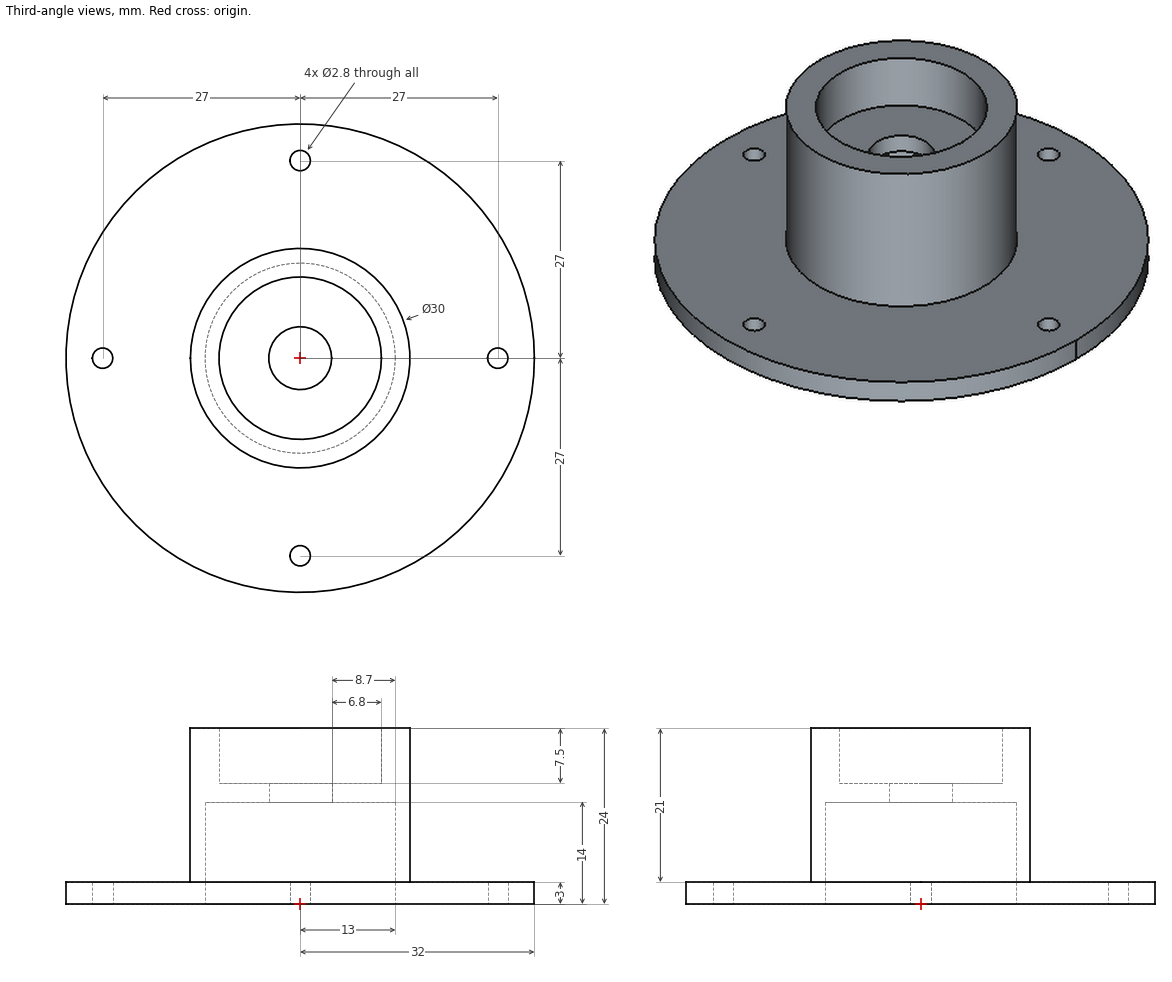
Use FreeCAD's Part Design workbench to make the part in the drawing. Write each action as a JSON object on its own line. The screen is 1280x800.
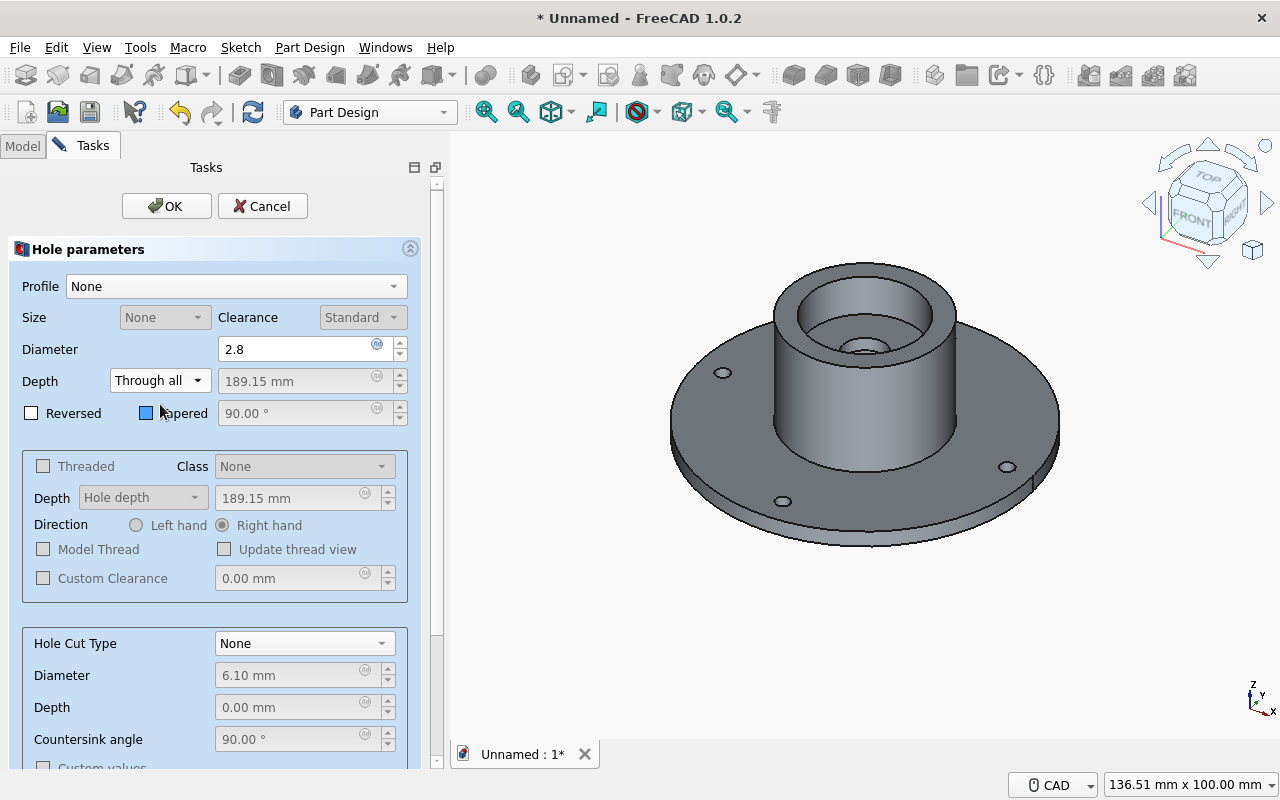
{"action": "left_click", "coordinate": [167, 206]}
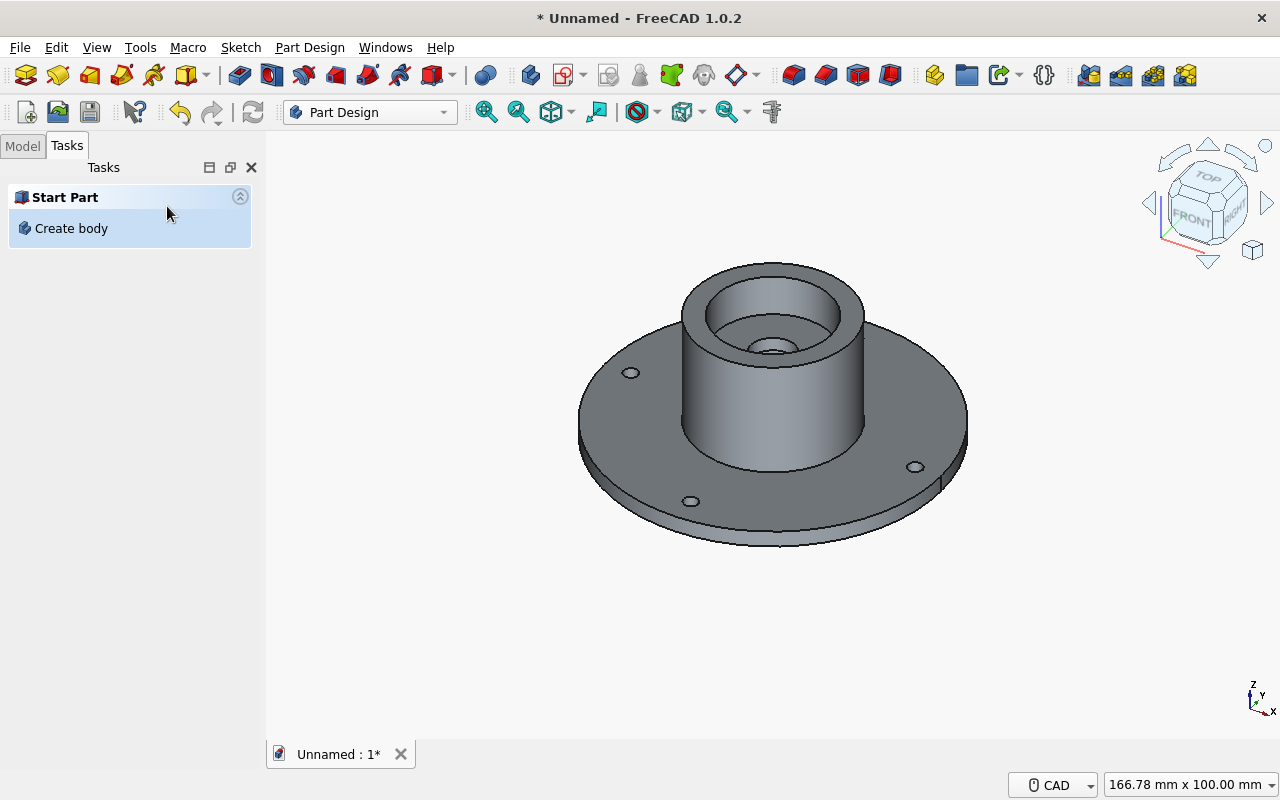
{"action": "key", "text": "0"}